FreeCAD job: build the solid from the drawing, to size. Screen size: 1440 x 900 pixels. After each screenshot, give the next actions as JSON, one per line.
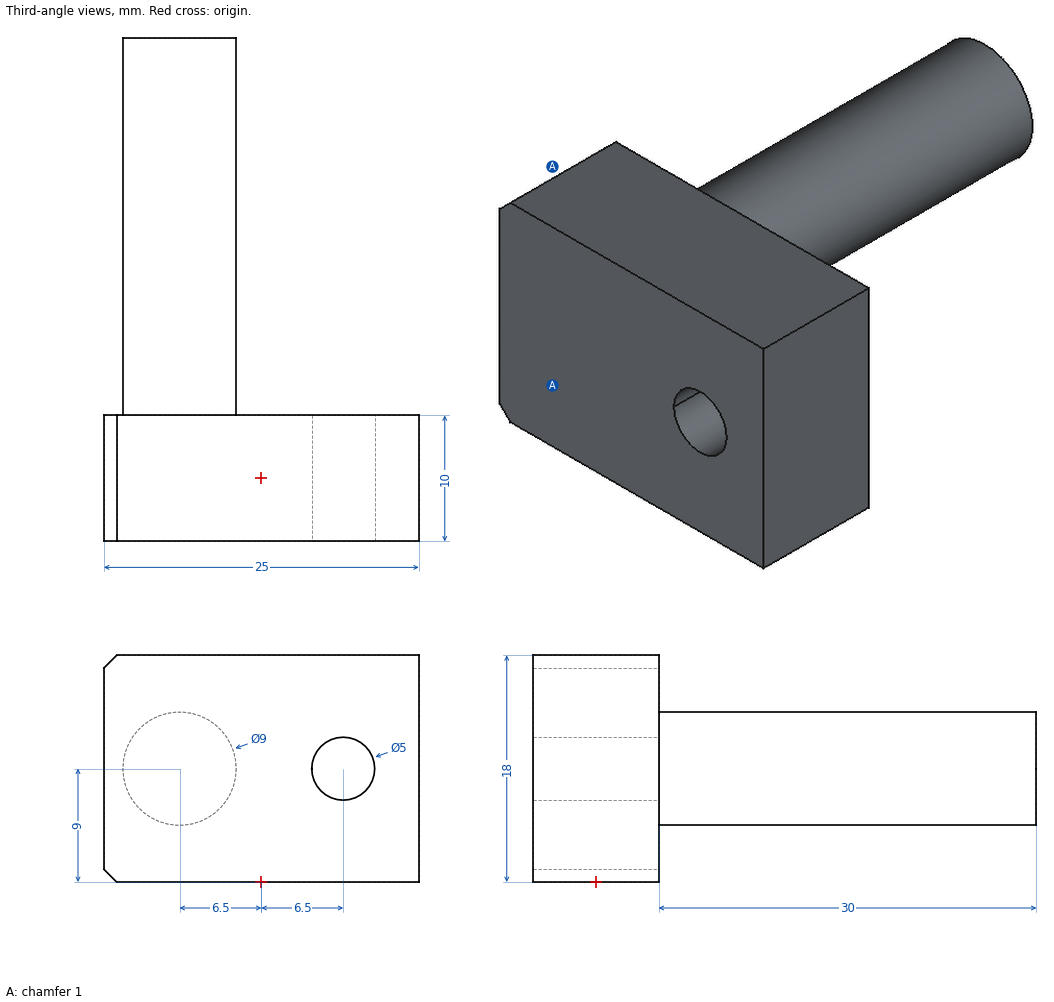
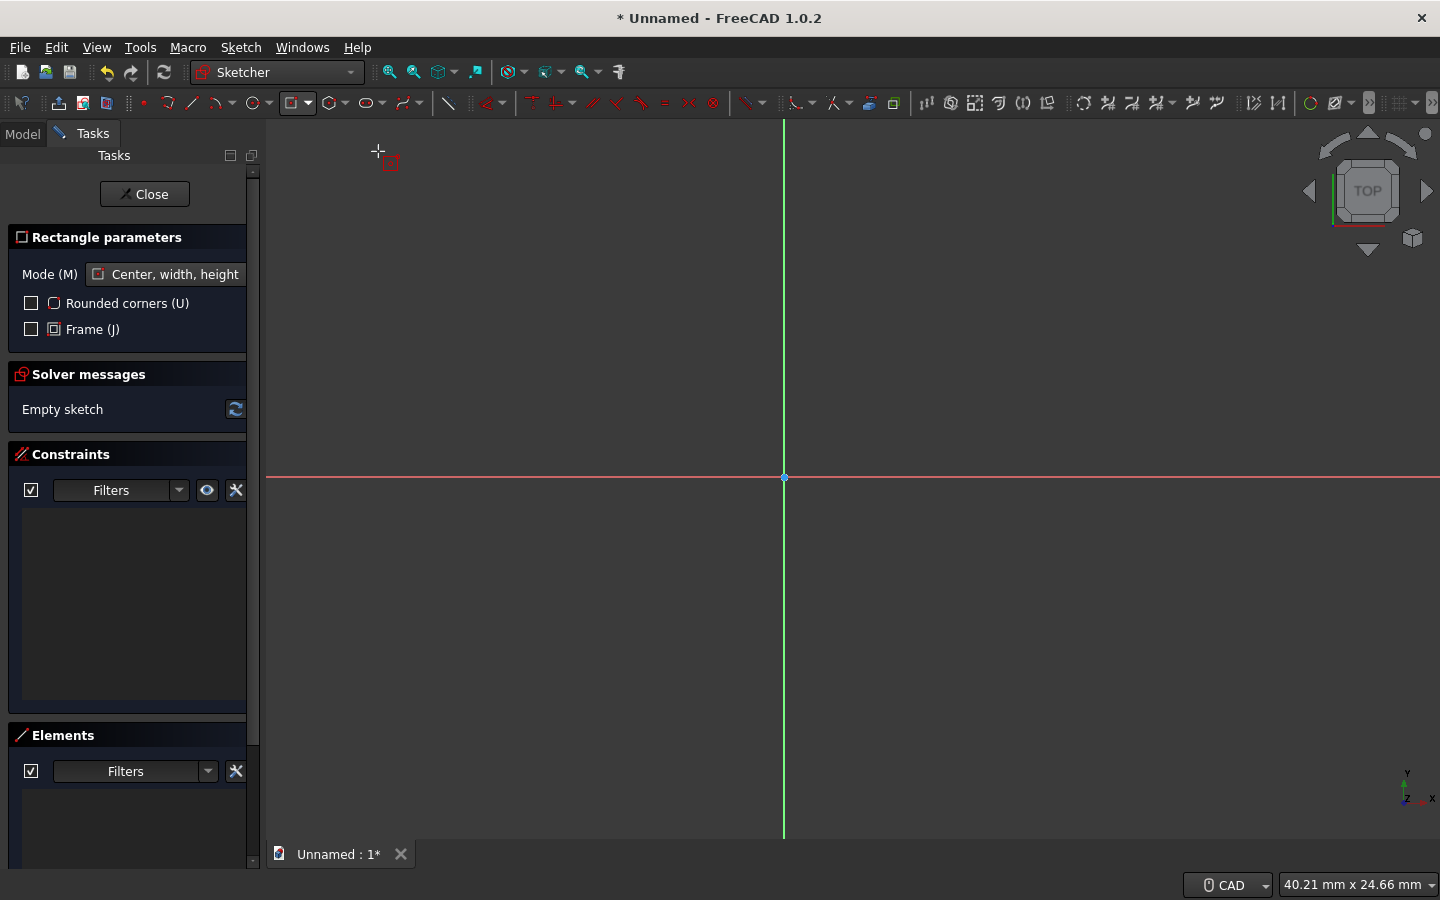
{"action": "left_click", "coordinate": [784, 477]}
{"action": "mouse_move", "coordinate": [1149, 331]}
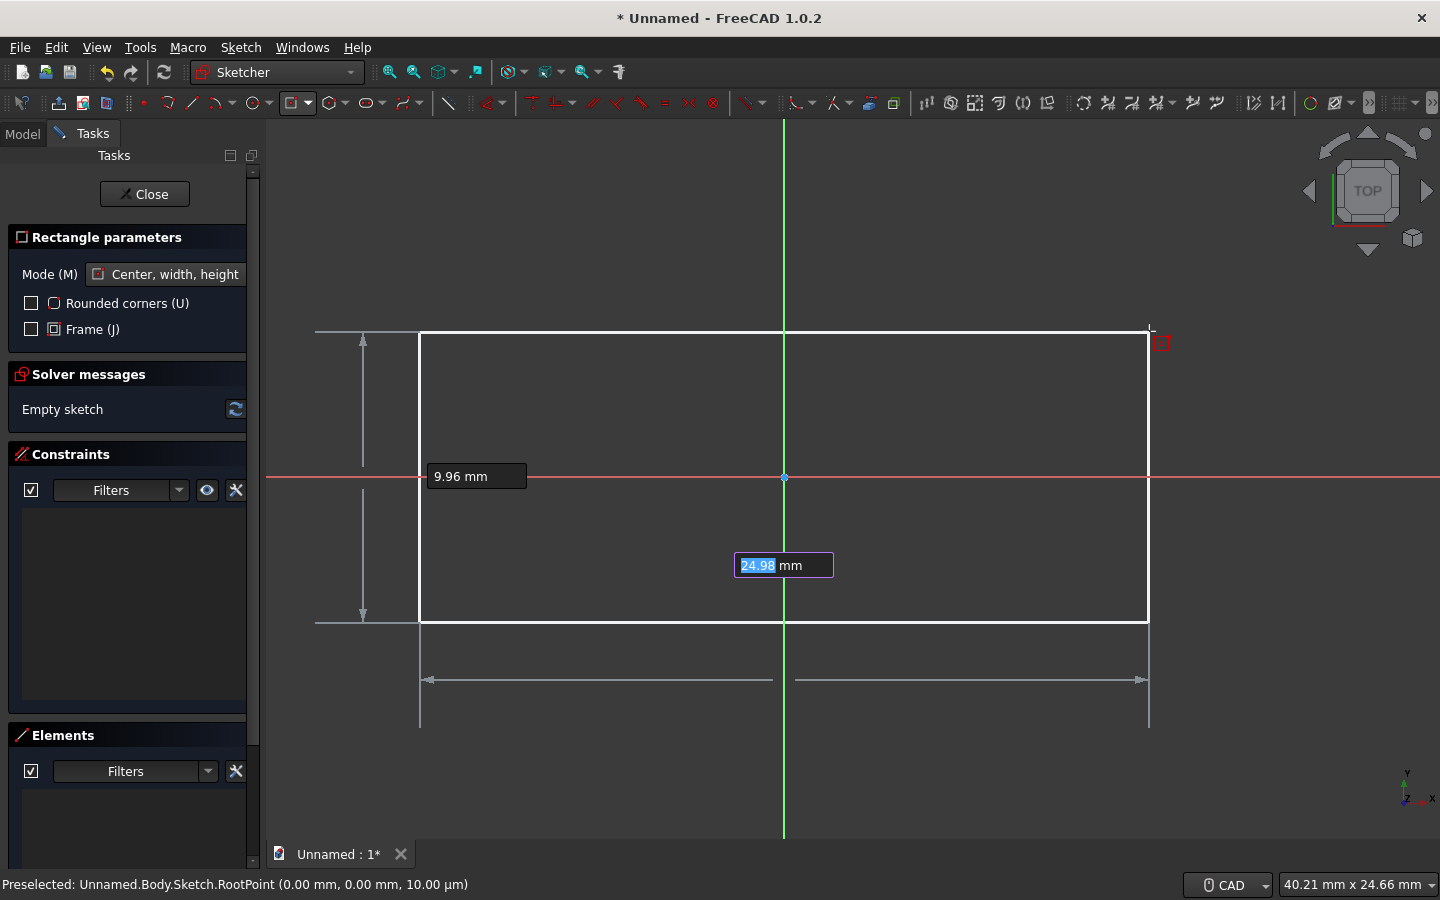
{"action": "type", "text": "25"}
{"action": "key", "text": "Tab"}
{"action": "type", "text": "10"}
{"action": "key", "text": "Return"}
{"action": "key", "text": "Escape"}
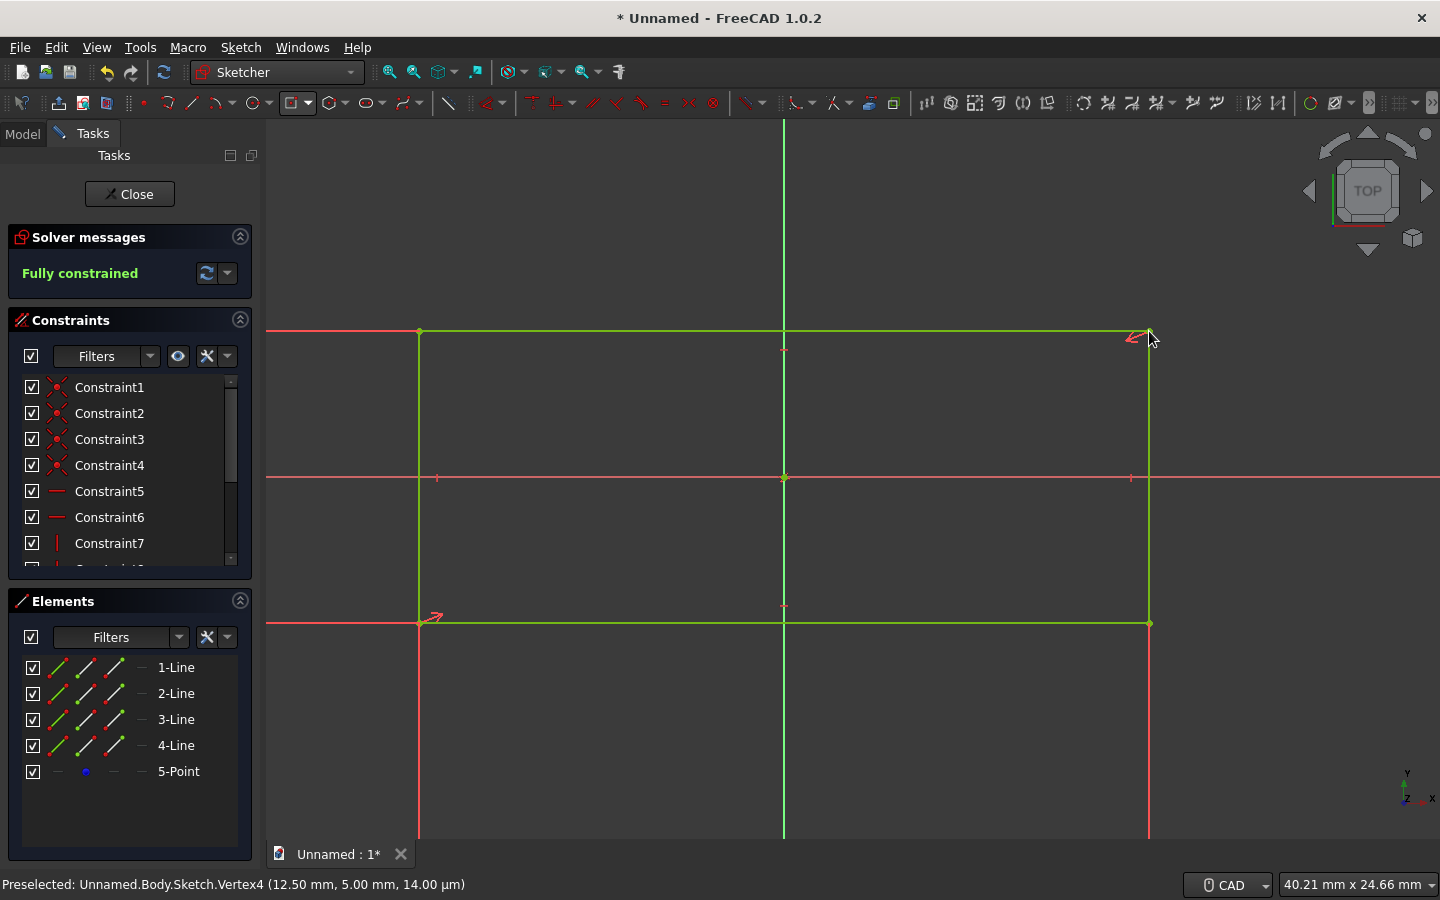
{"action": "left_click", "coordinate": [130, 194]}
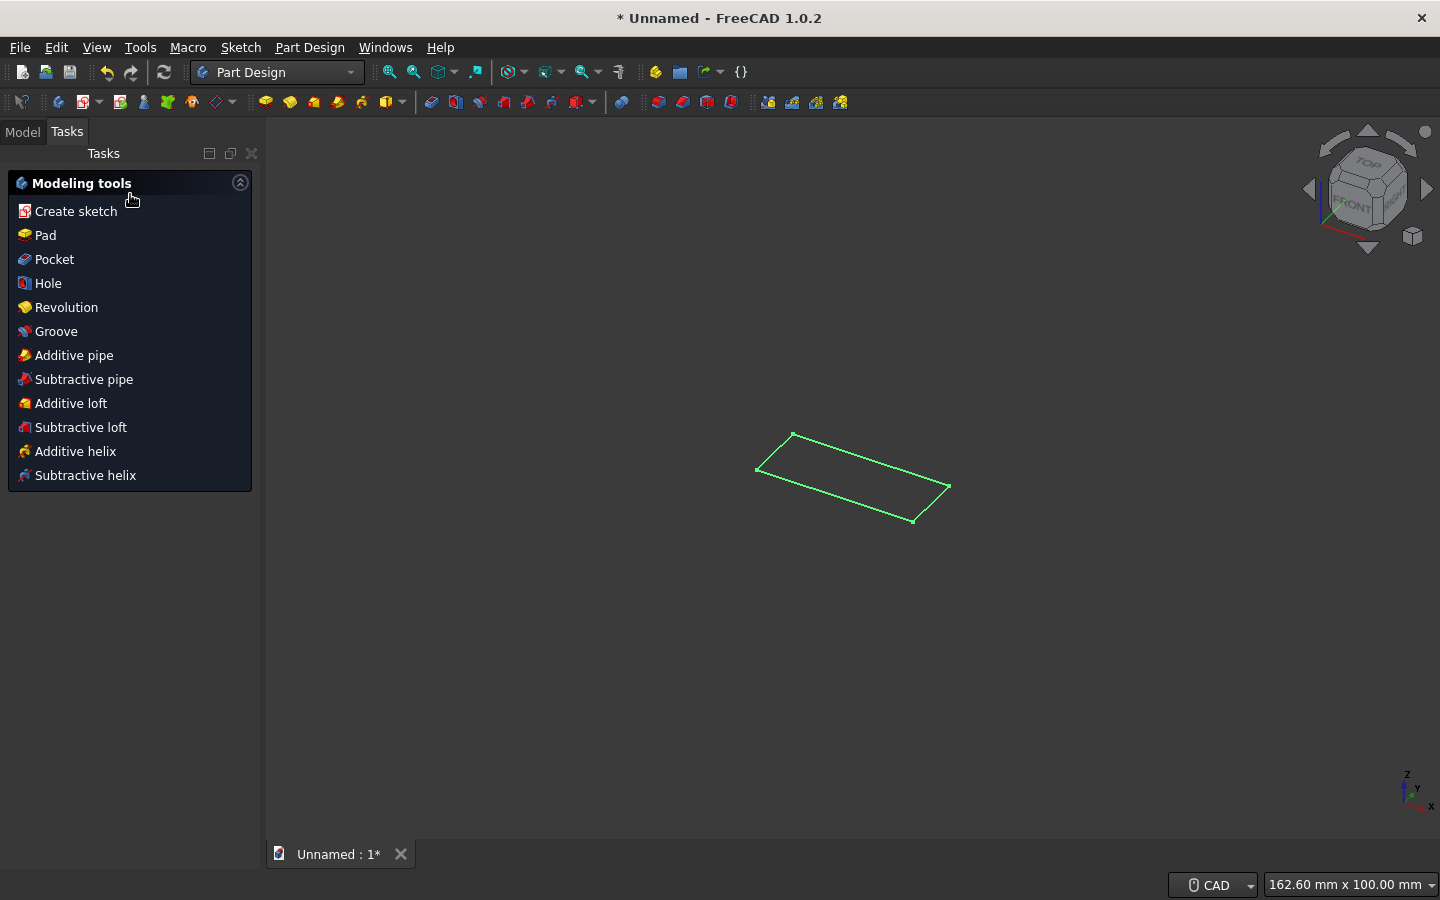
{"action": "left_click", "coordinate": [266, 102]}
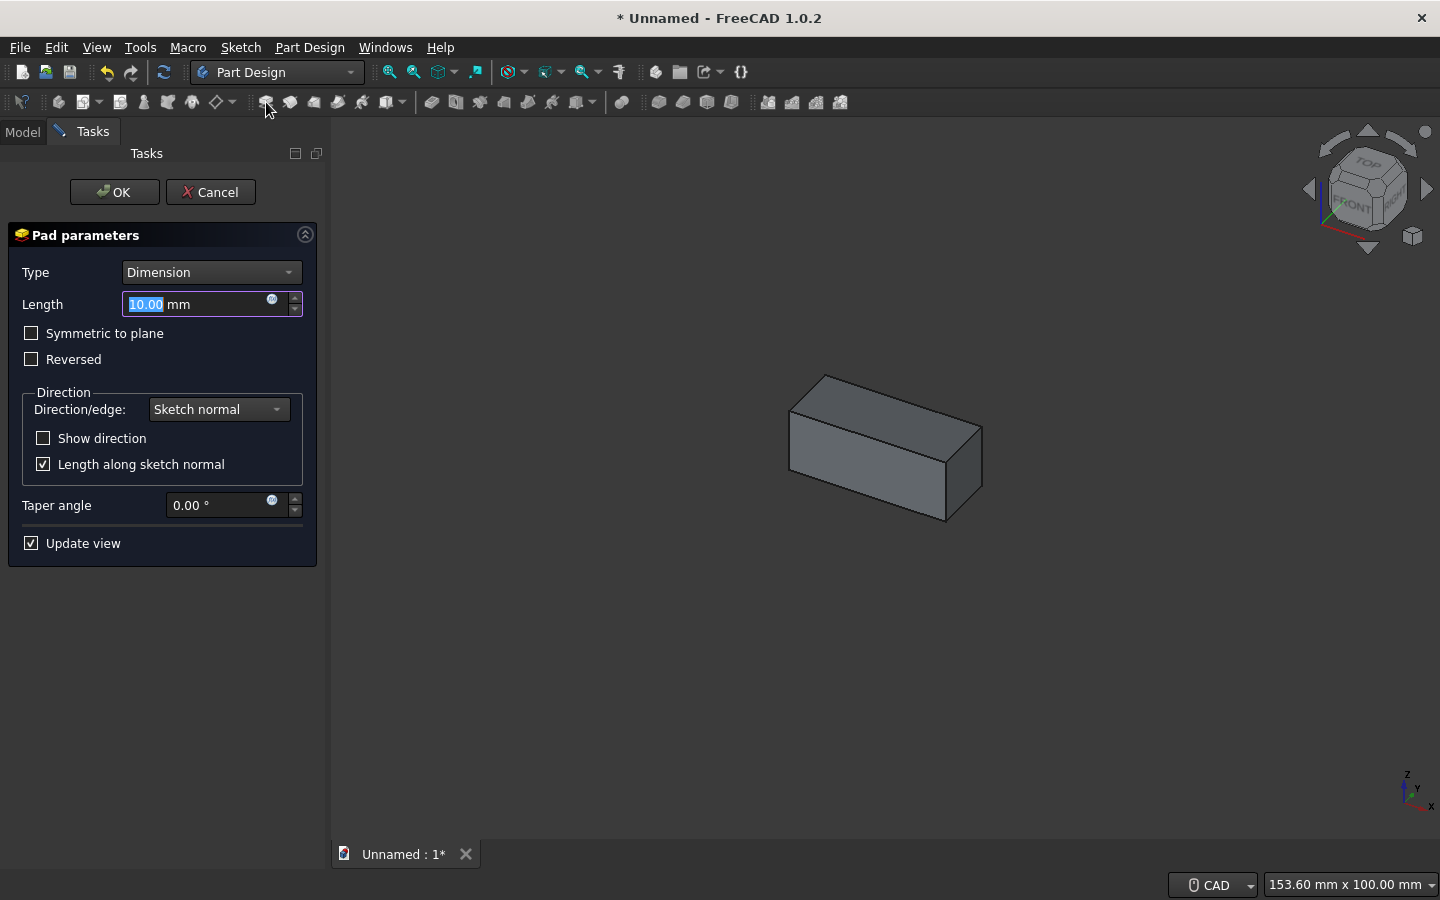
{"action": "type", "text": "18"}
{"action": "key", "text": "Tab"}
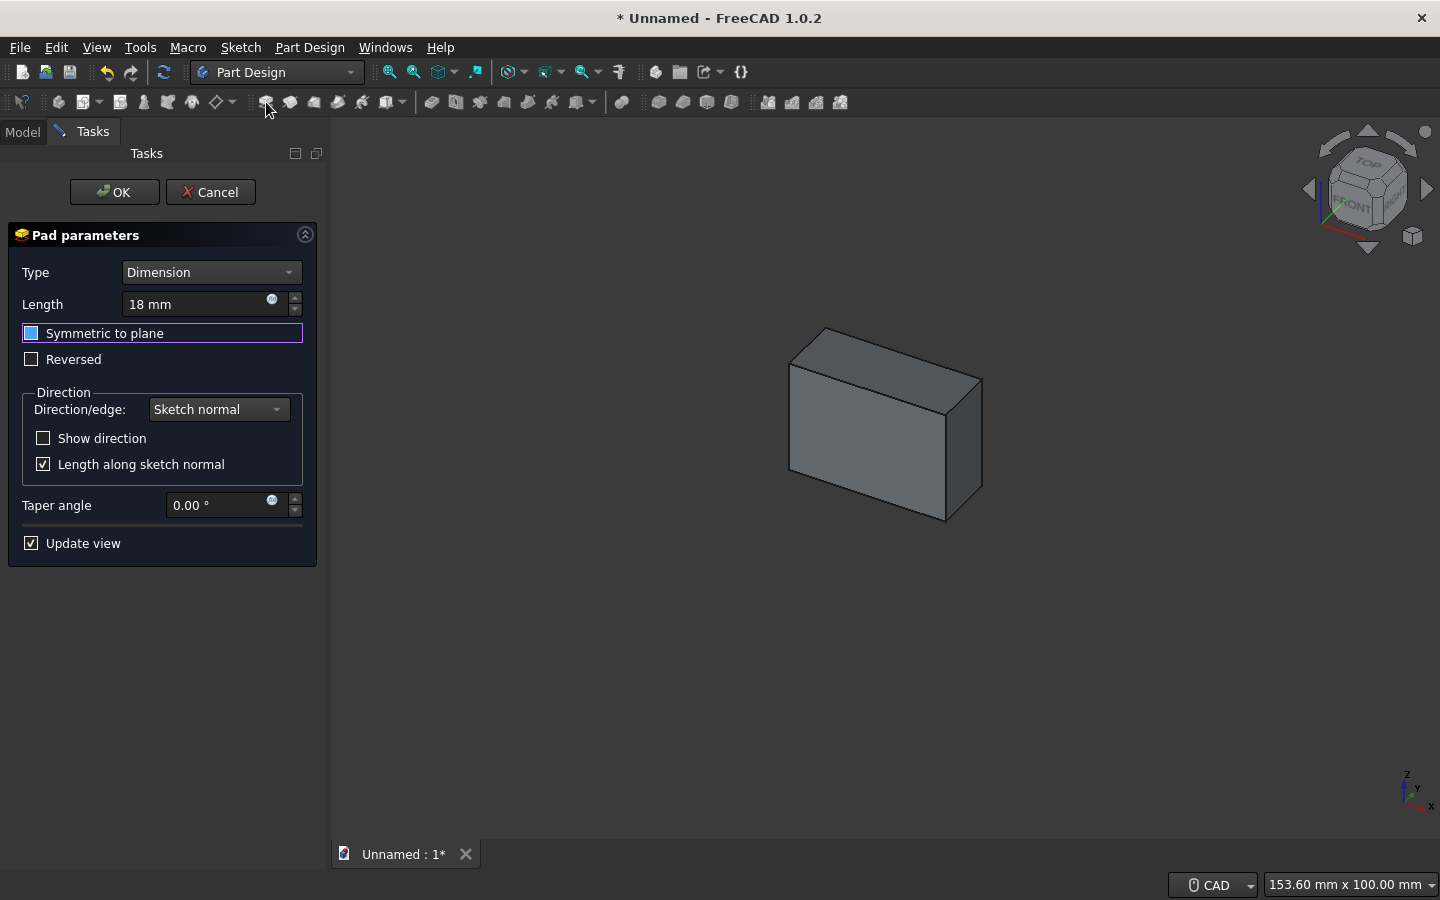
{"action": "left_click", "coordinate": [115, 192]}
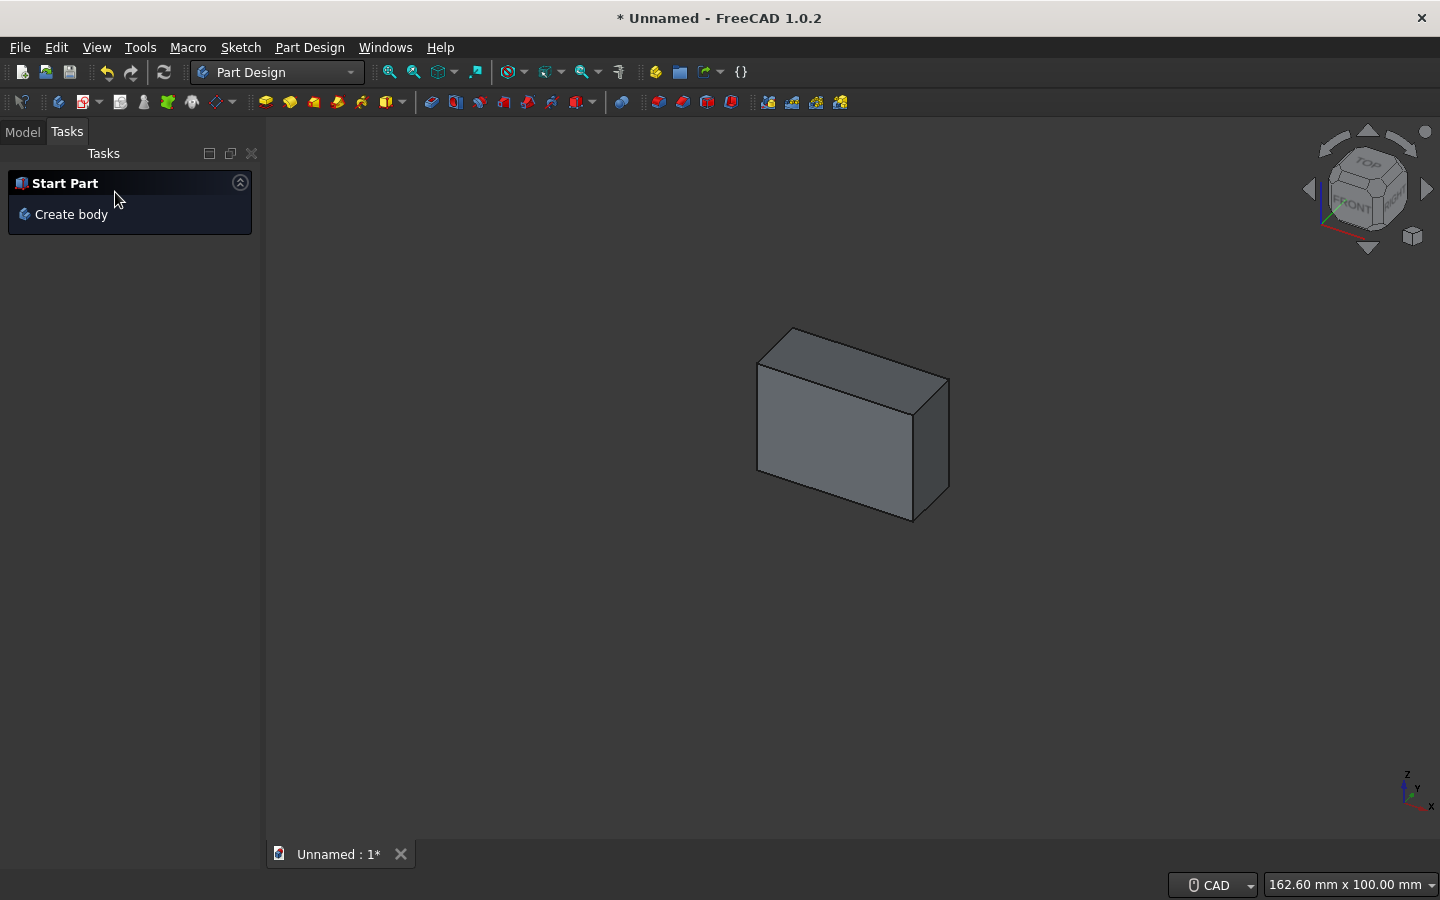
{"action": "key", "text": "v f"}